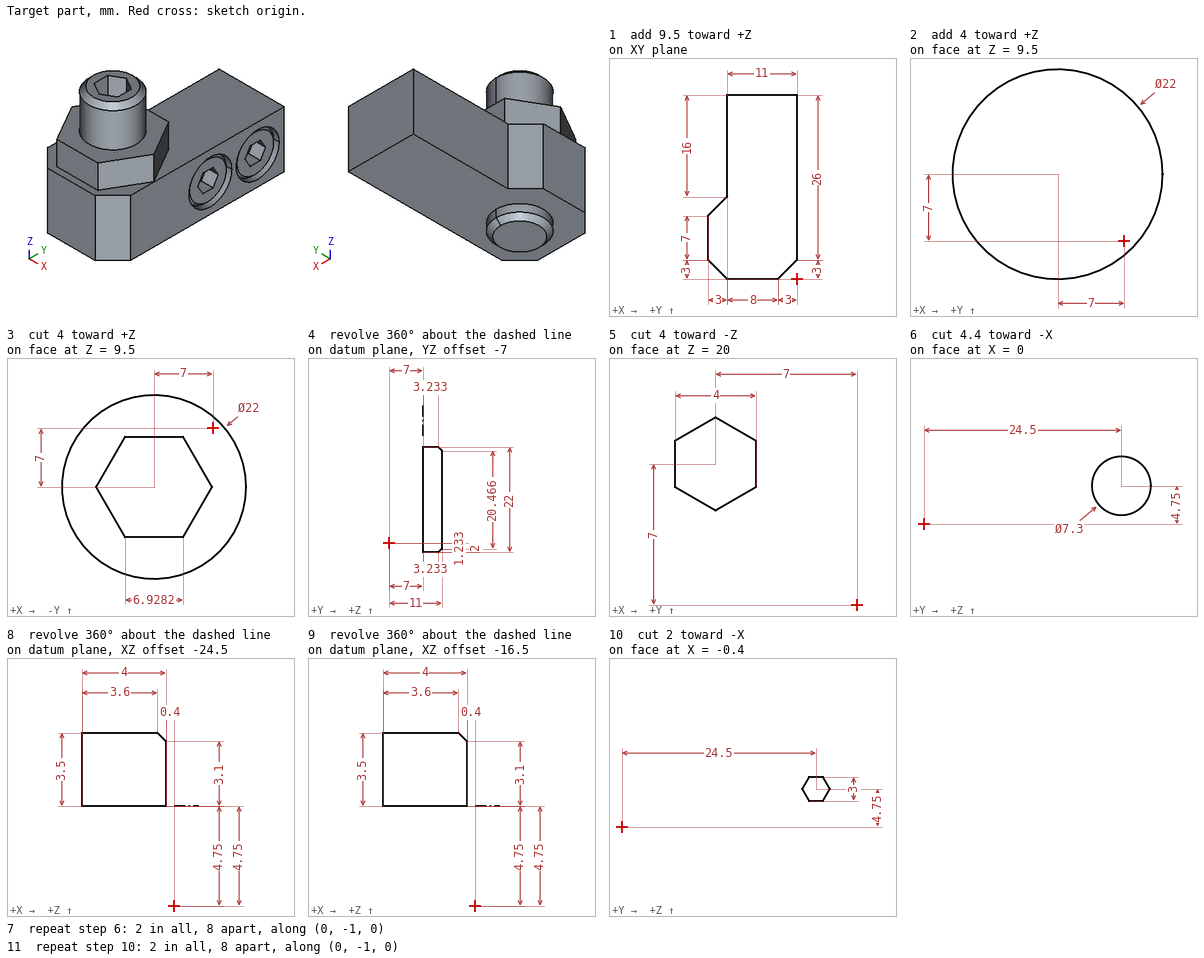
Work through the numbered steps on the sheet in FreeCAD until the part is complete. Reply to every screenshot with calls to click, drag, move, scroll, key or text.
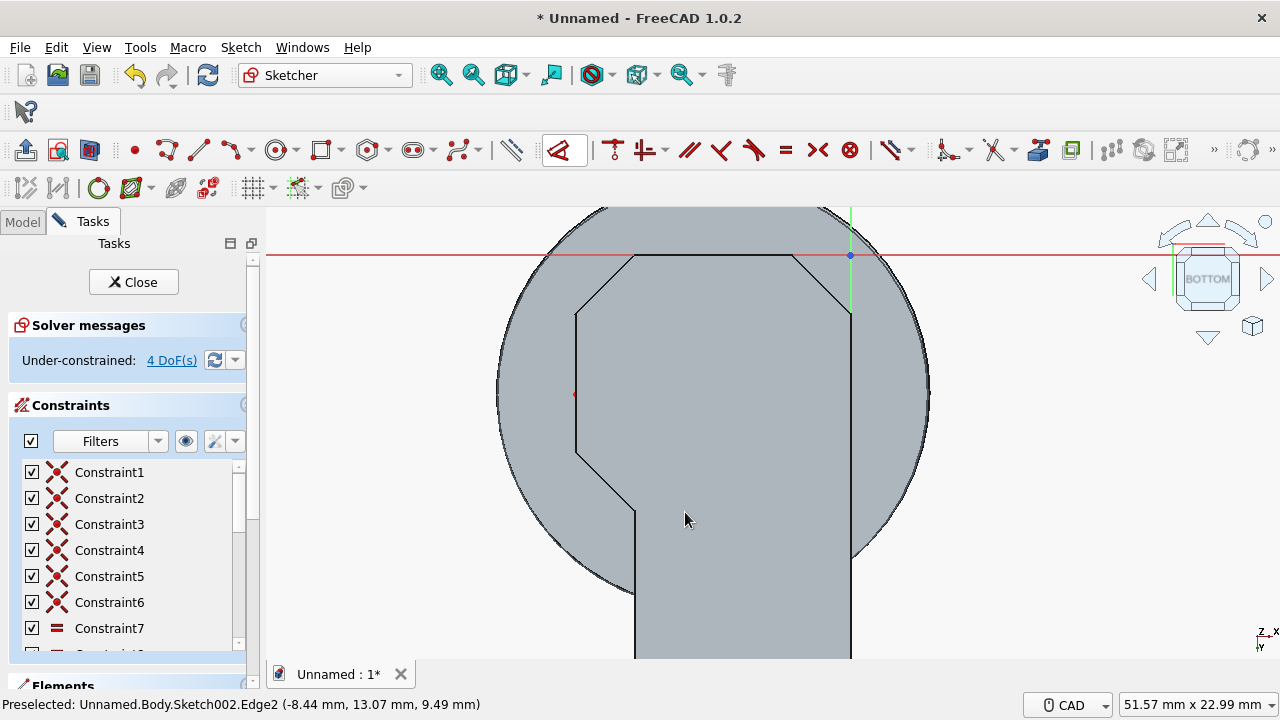
click(864, 242)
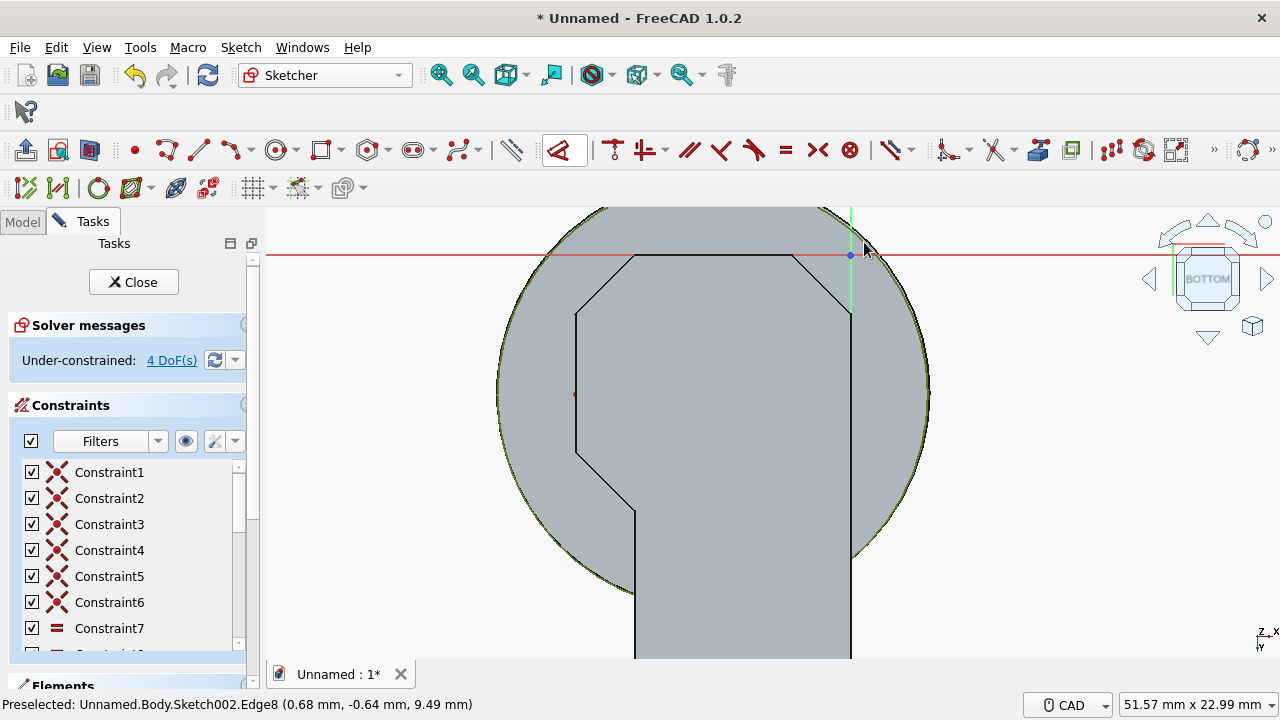
key(k)
key(o)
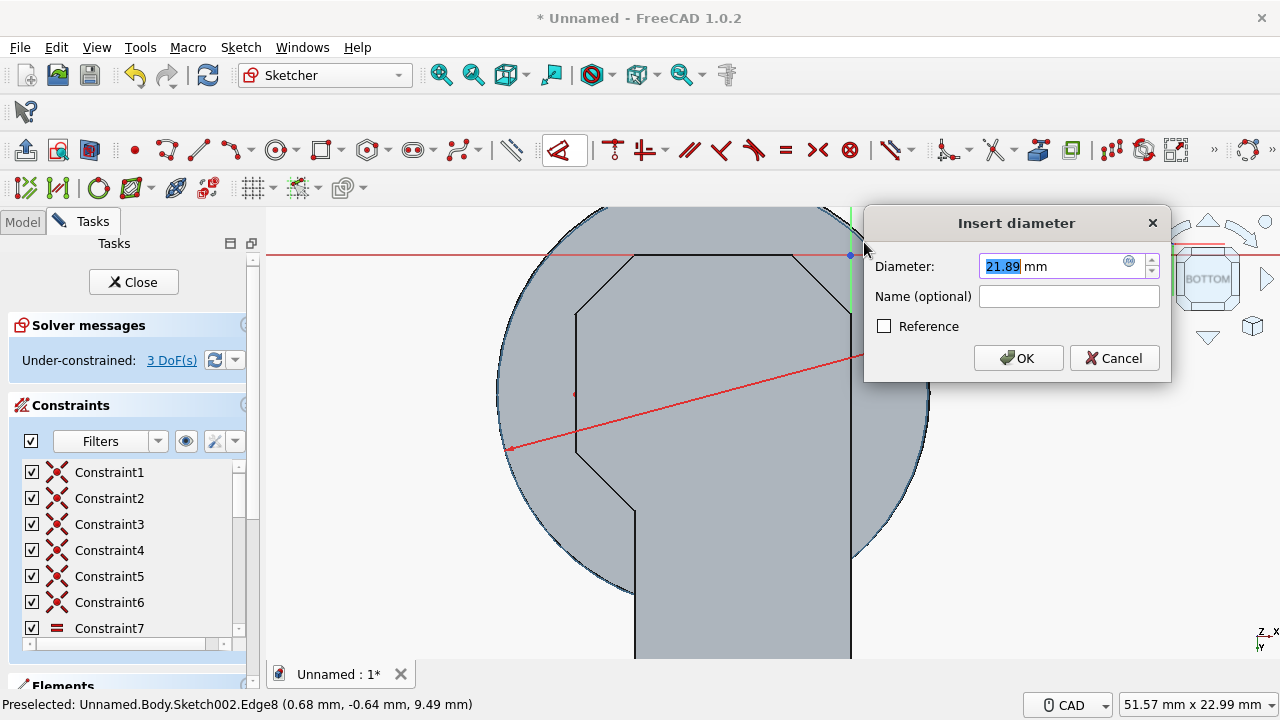
text(22)
key(Return)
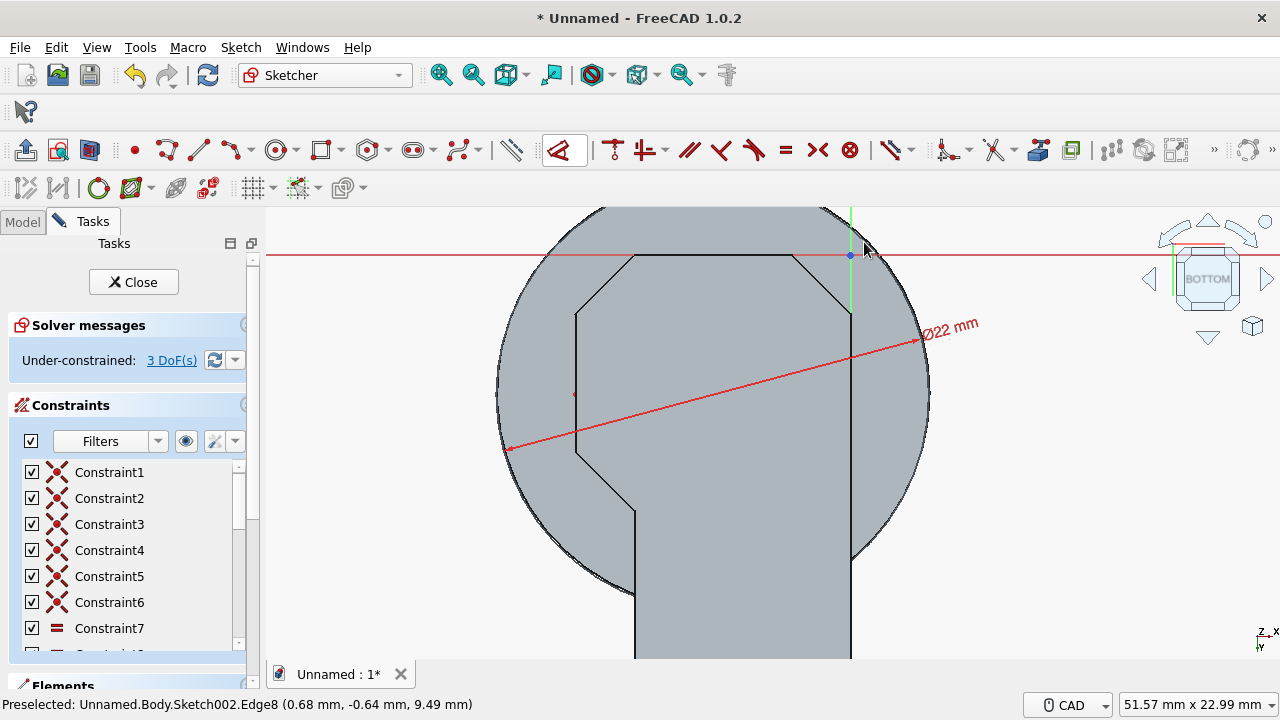
click(713, 395)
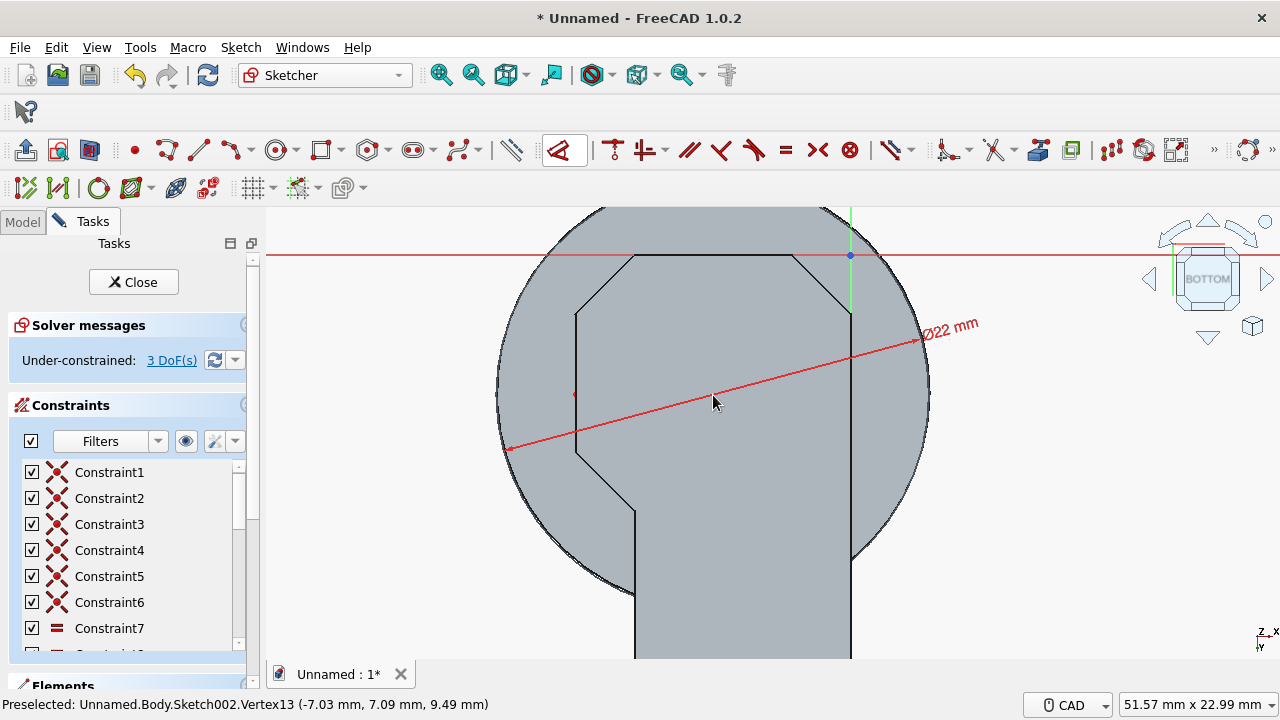
key(l)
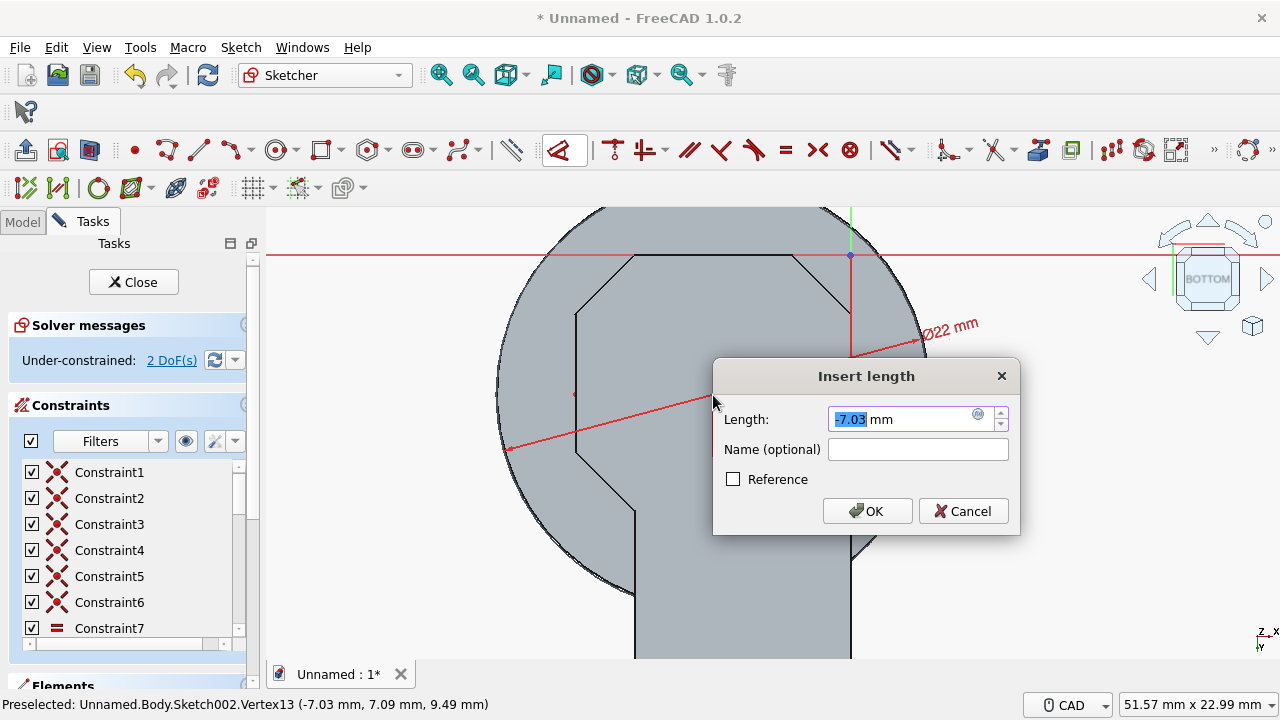
text(-7)
key(Return)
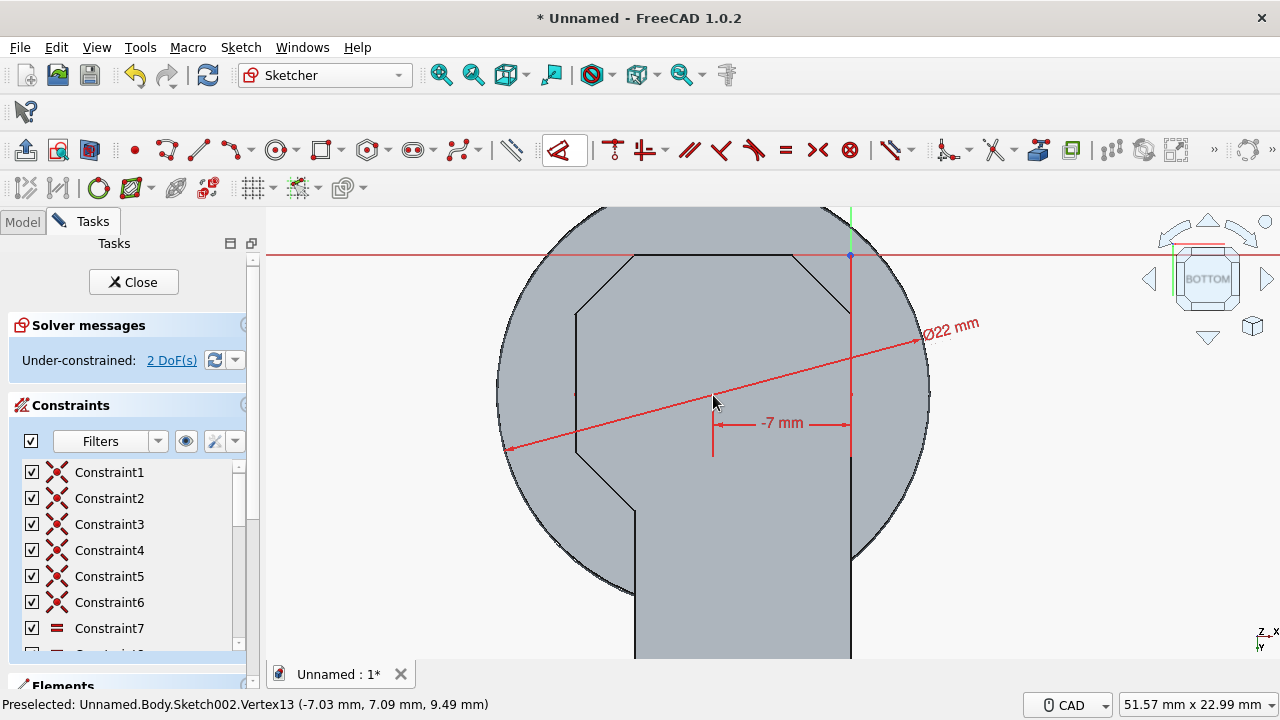
click(713, 395)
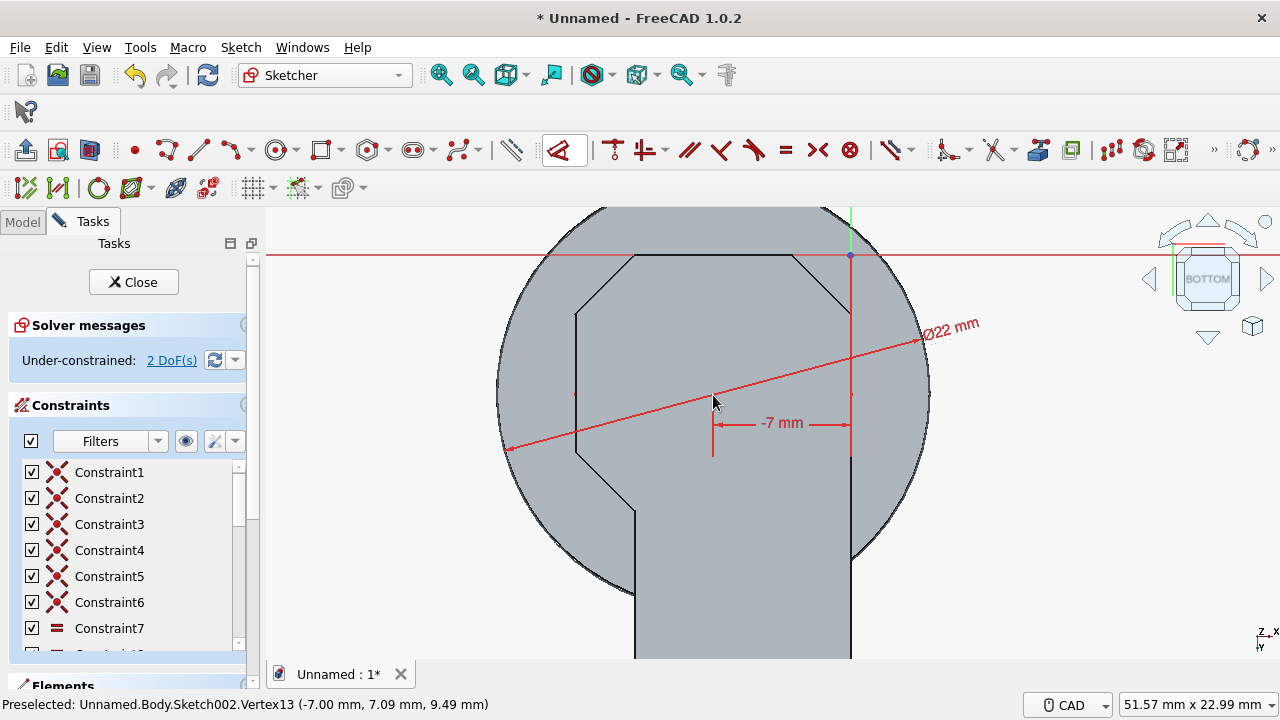
key(i)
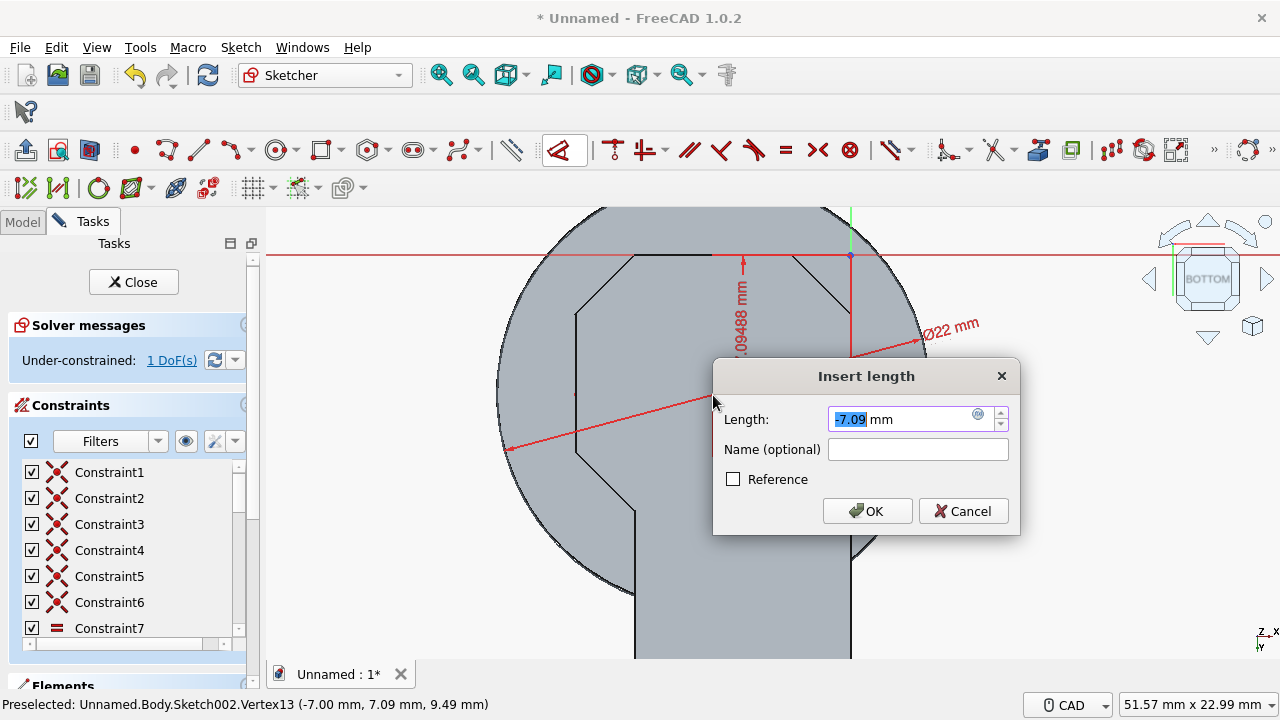
text(-7)
key(Return)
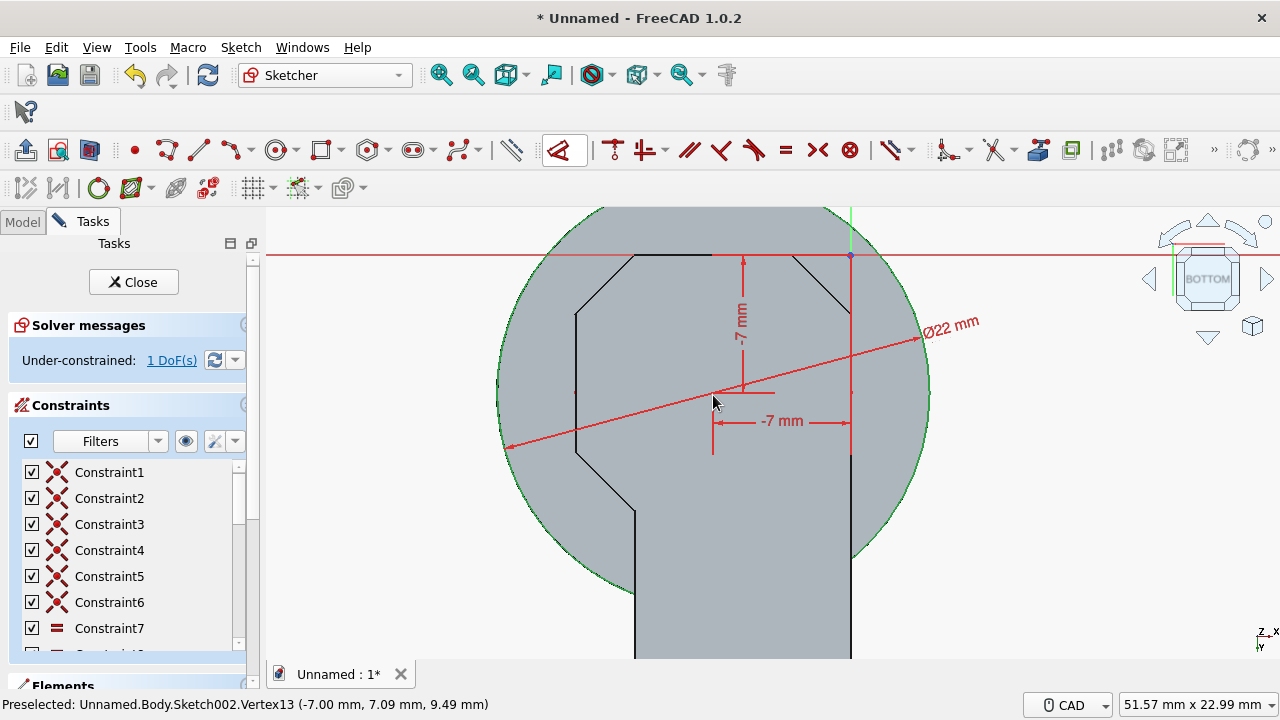
click(686, 511)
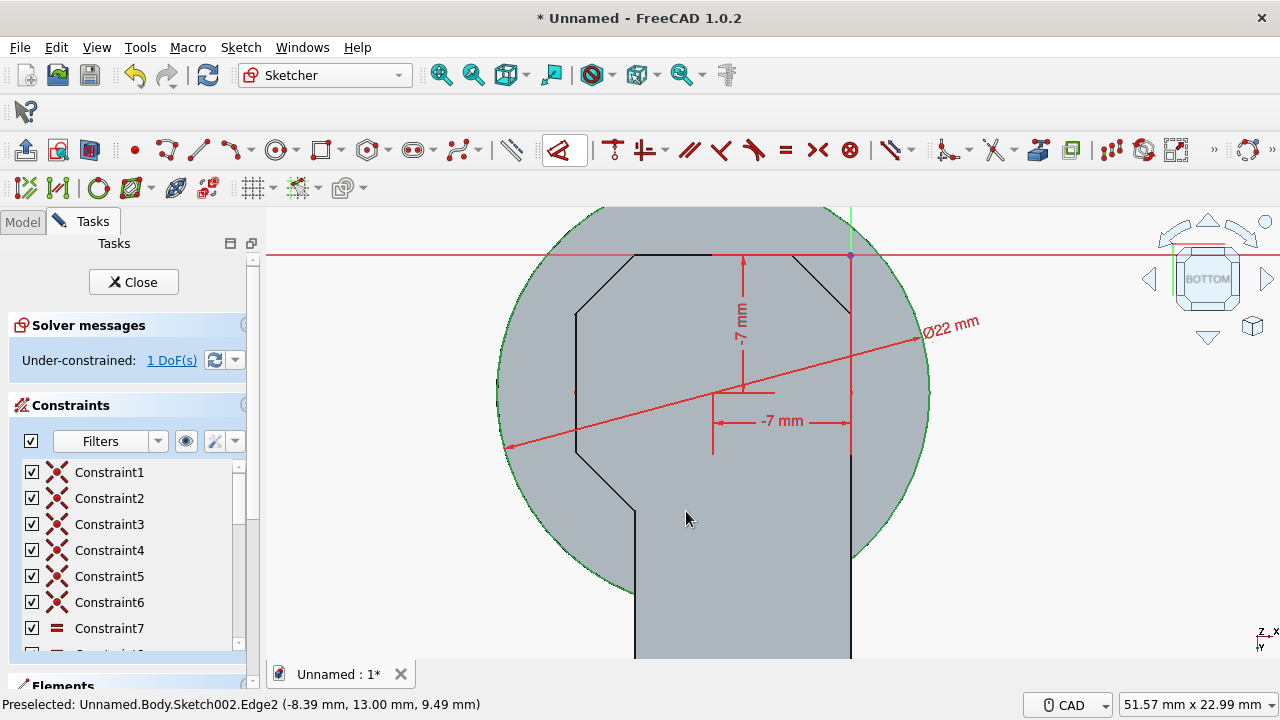
key(l)